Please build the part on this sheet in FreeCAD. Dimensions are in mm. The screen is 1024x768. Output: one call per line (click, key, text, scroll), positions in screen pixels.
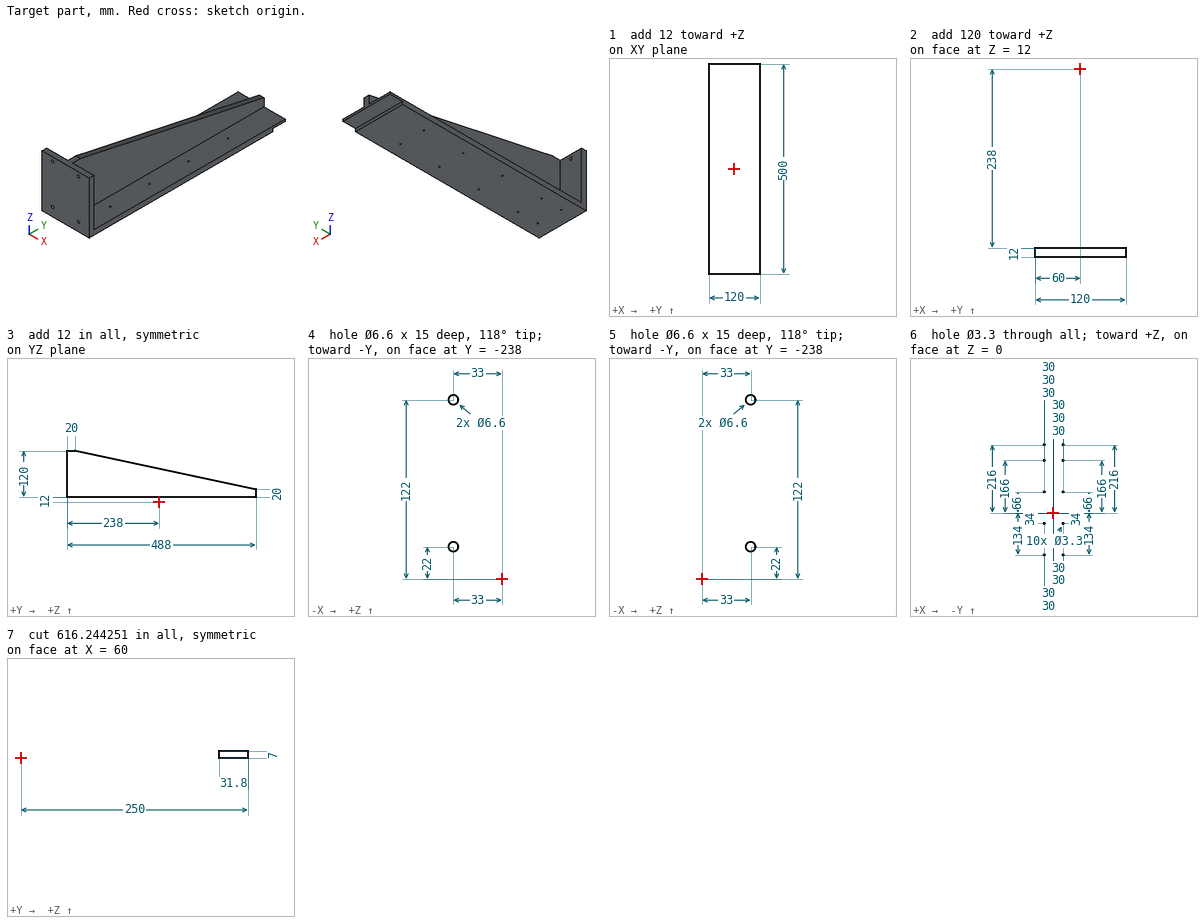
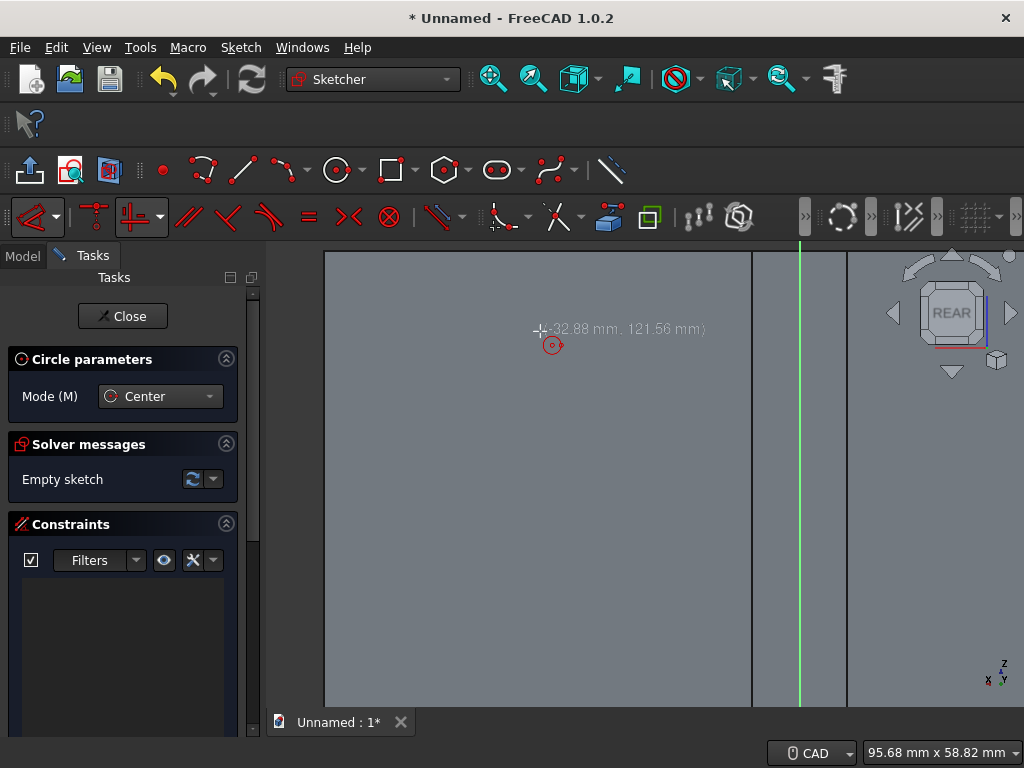
click(538, 330)
click(557, 312)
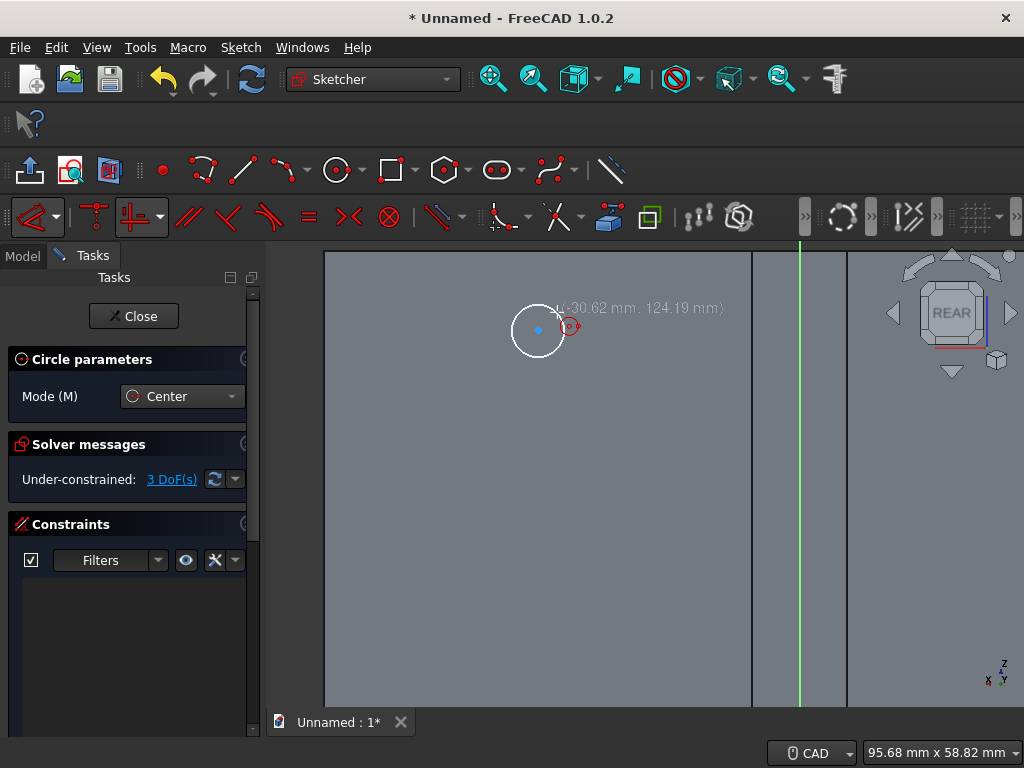
scroll(542, 333, down, 6)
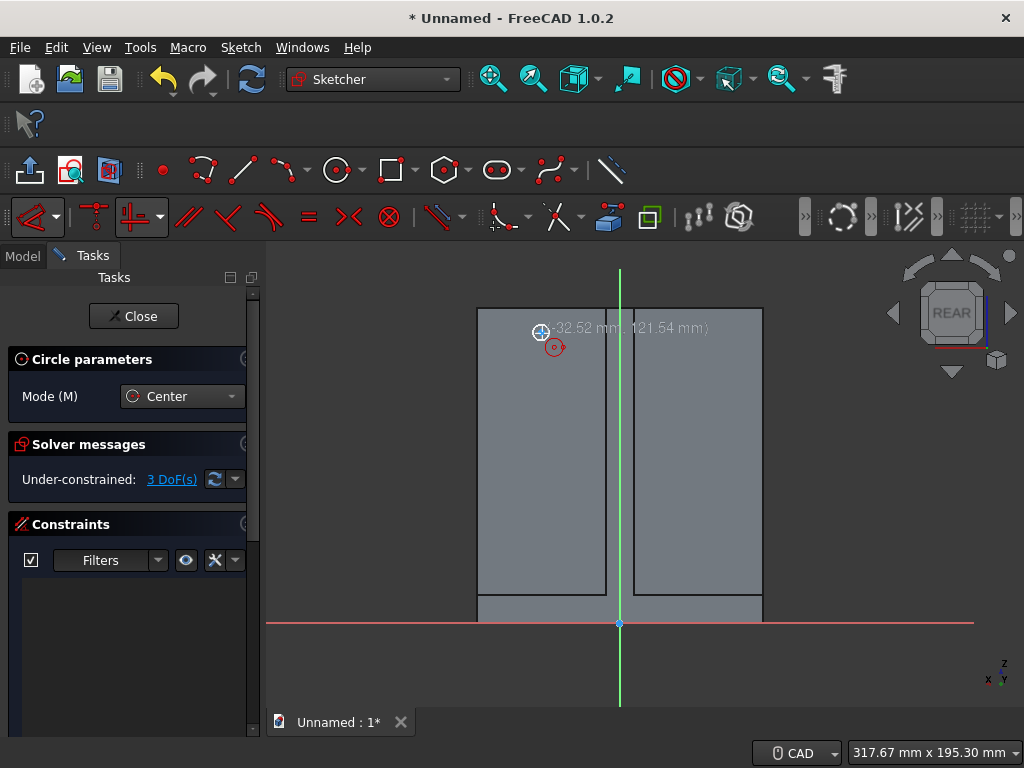
scroll(541, 571, up, 6)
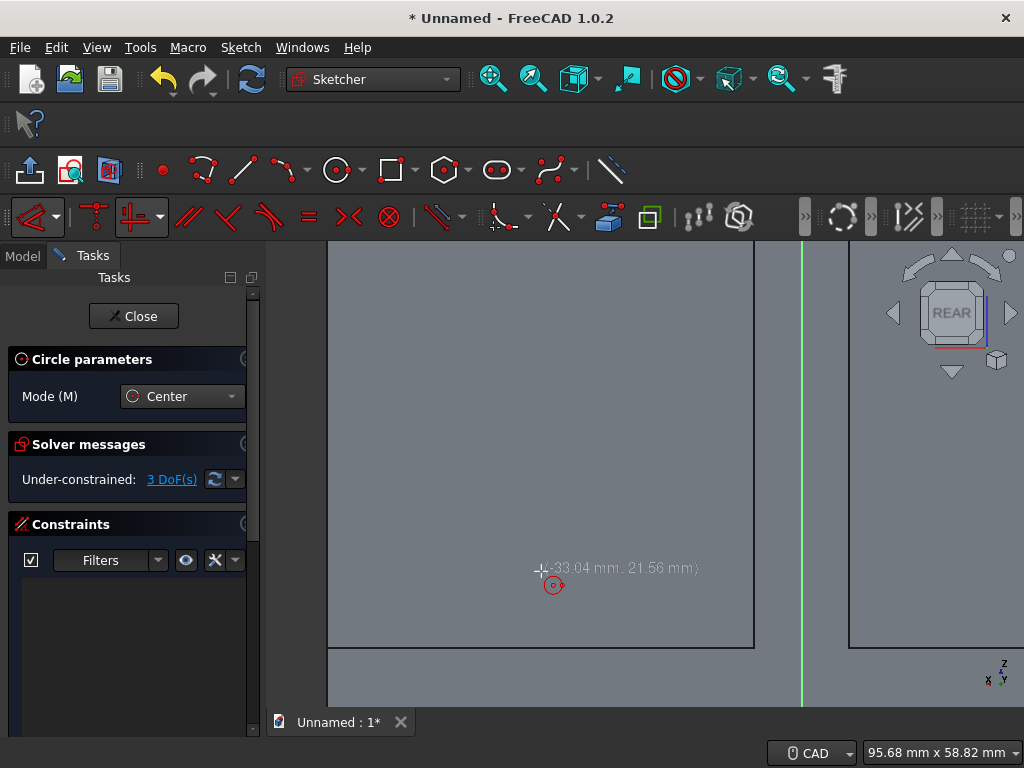
click(540, 569)
click(559, 551)
key(Escape)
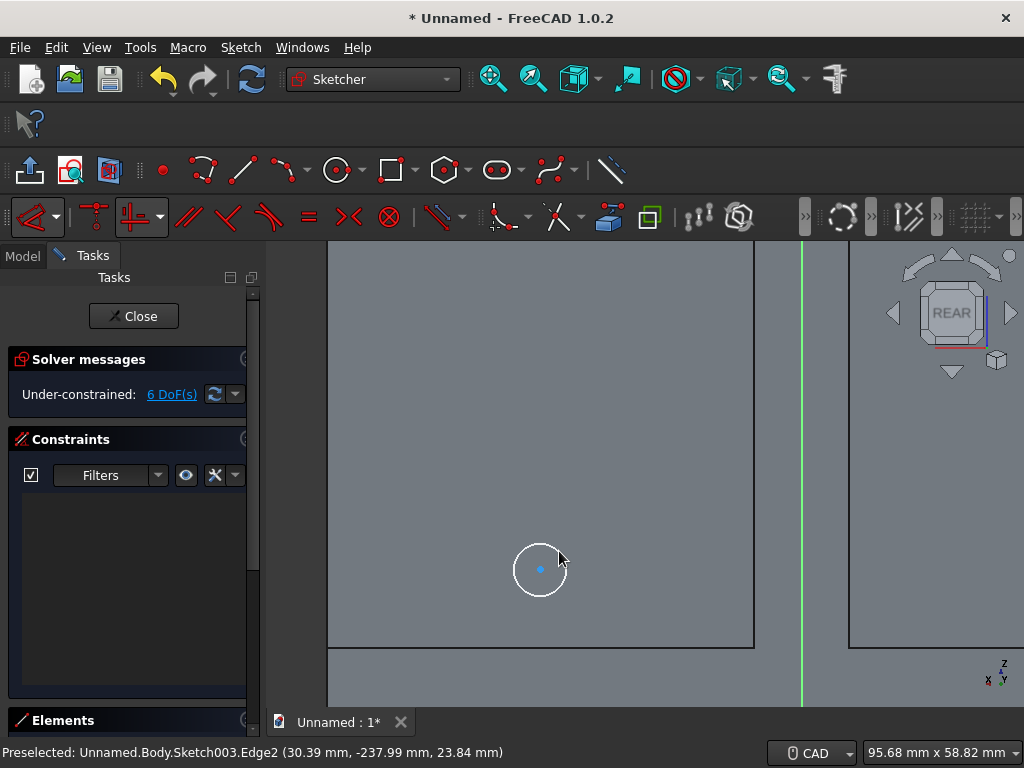
scroll(541, 572, down, 6)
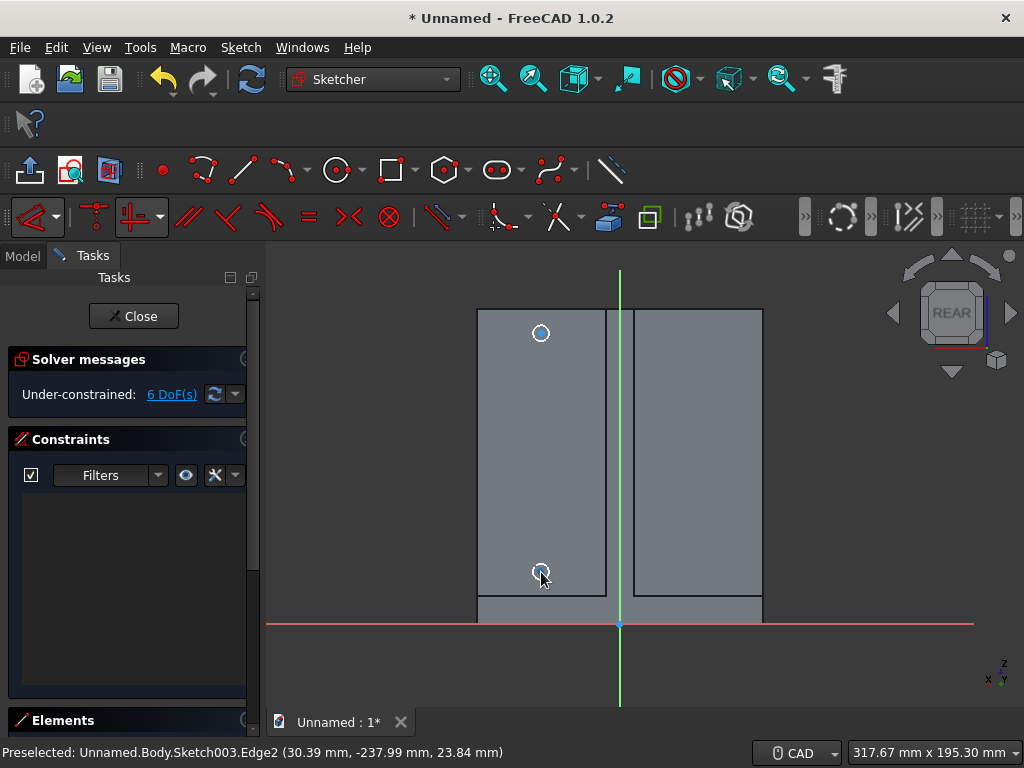
scroll(547, 328, up, 3)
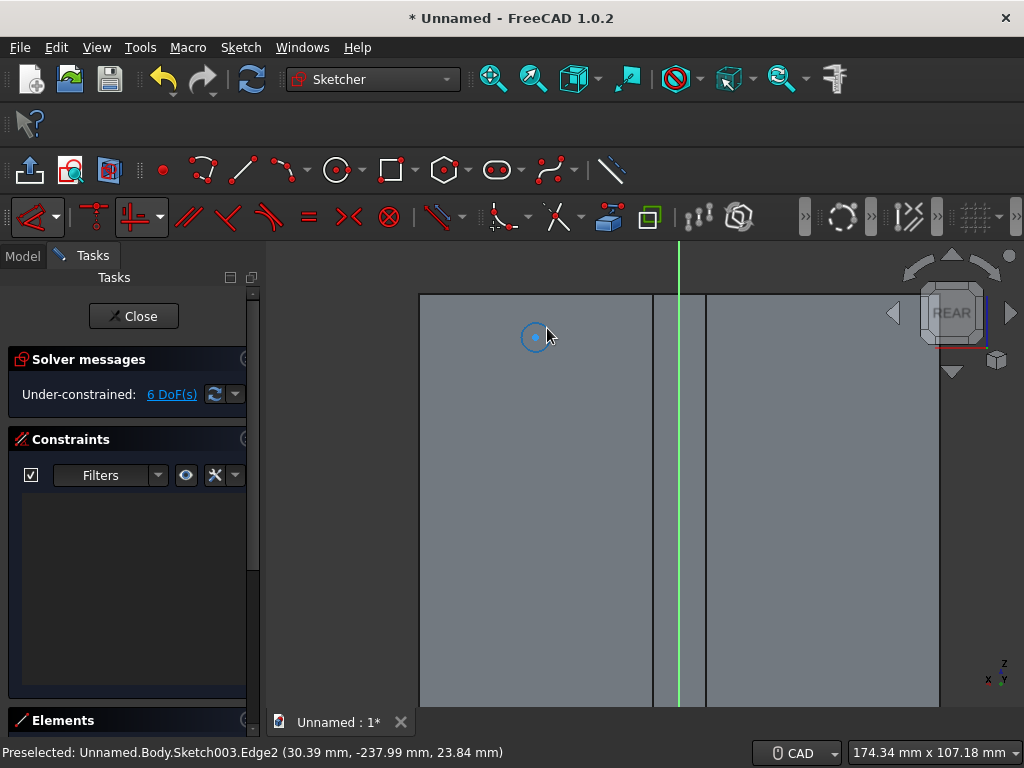
click(546, 327)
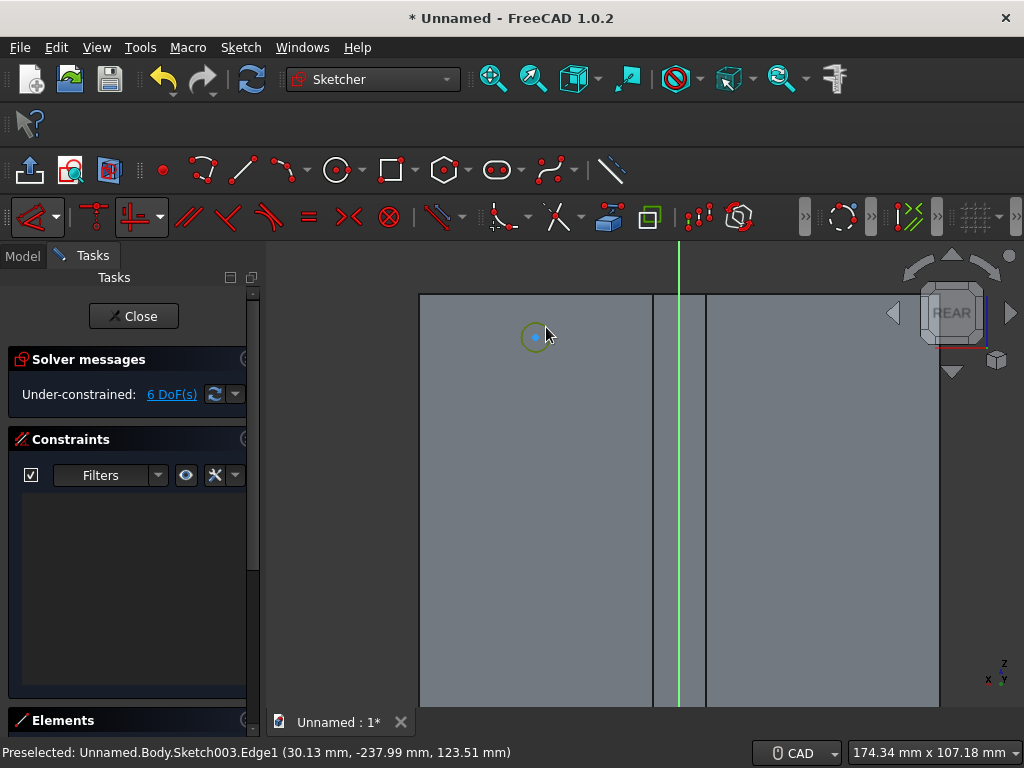
scroll(547, 327, down, 3)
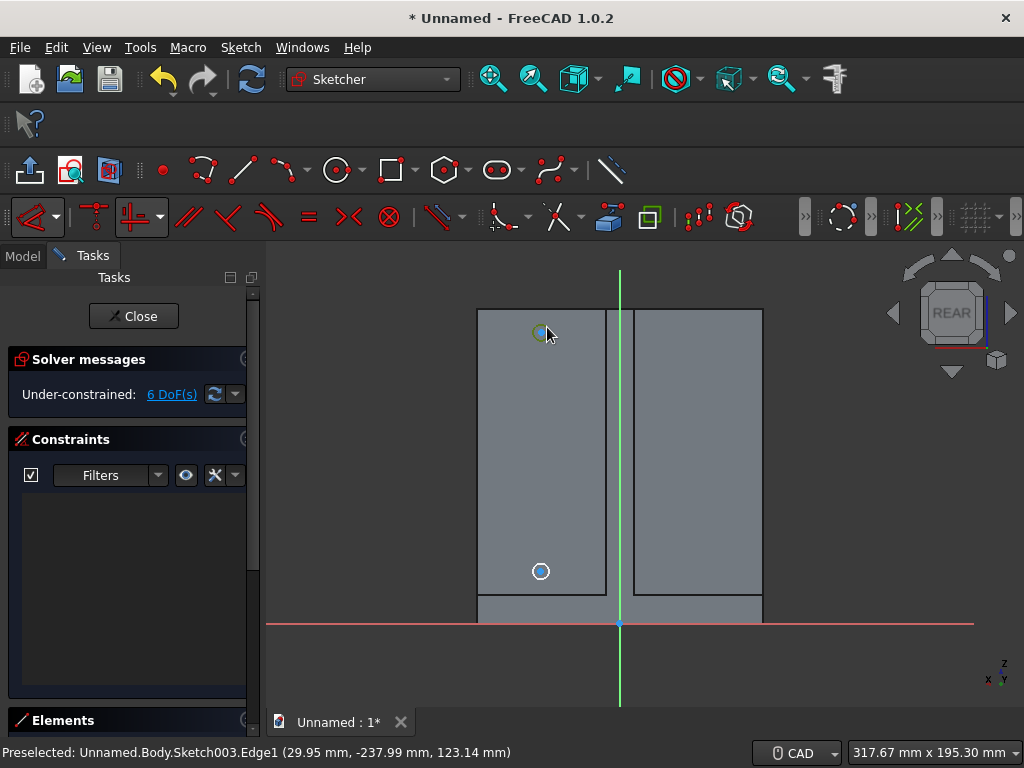
scroll(547, 566, up, 3)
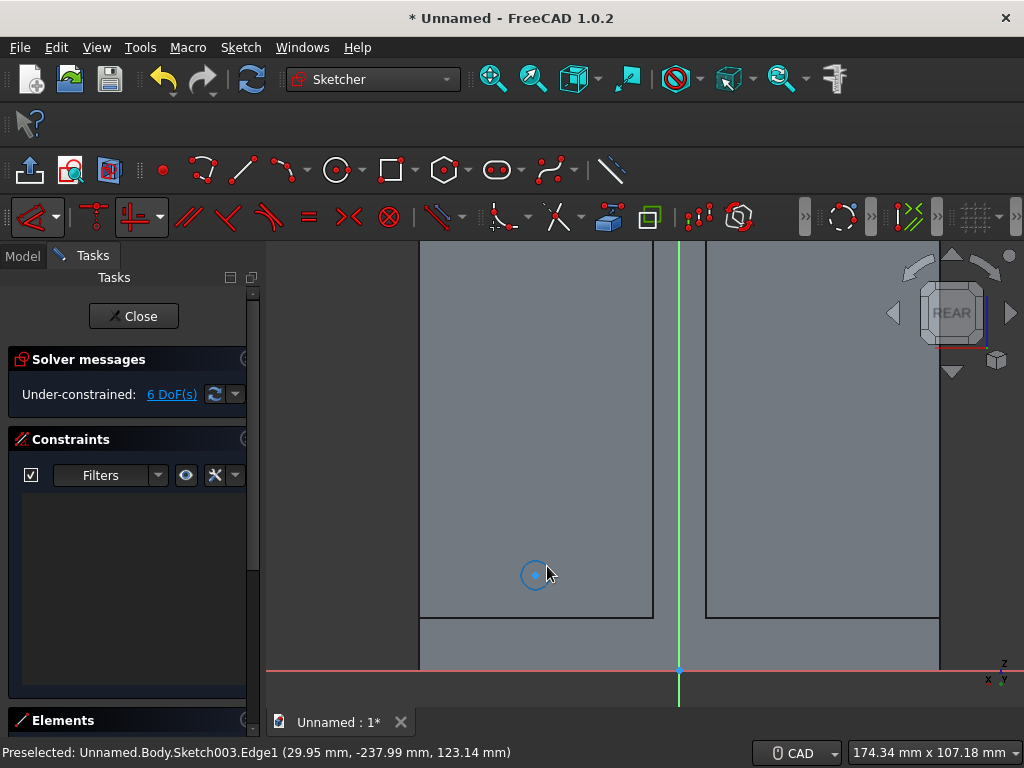
click(546, 565)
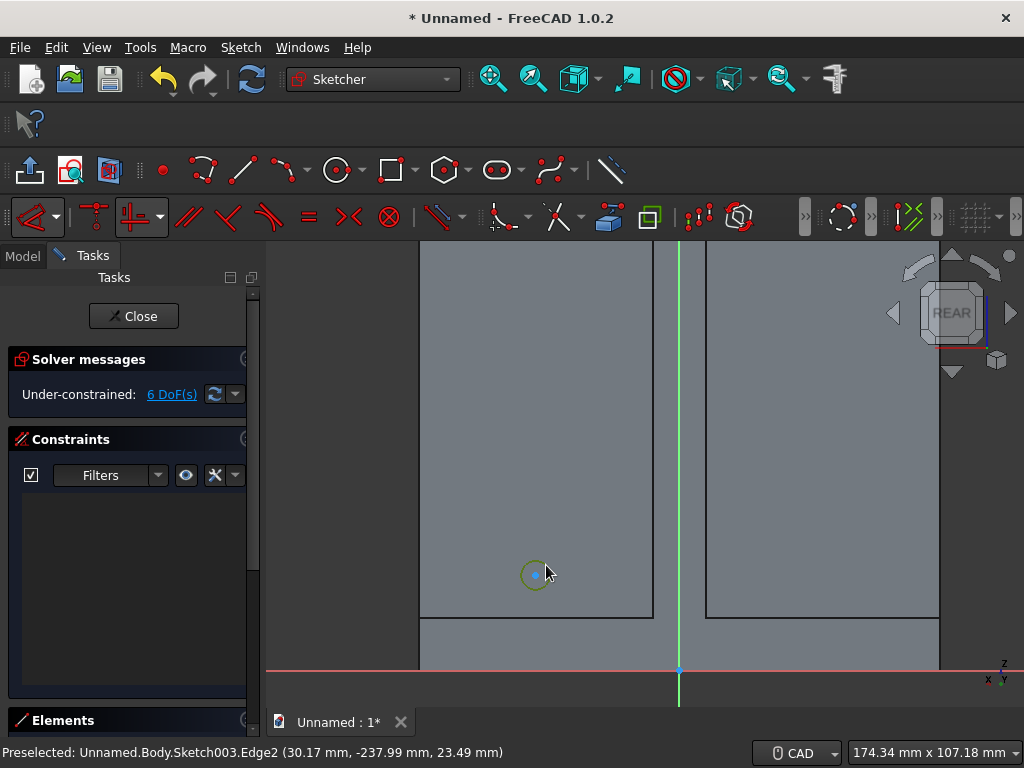
click(310, 218)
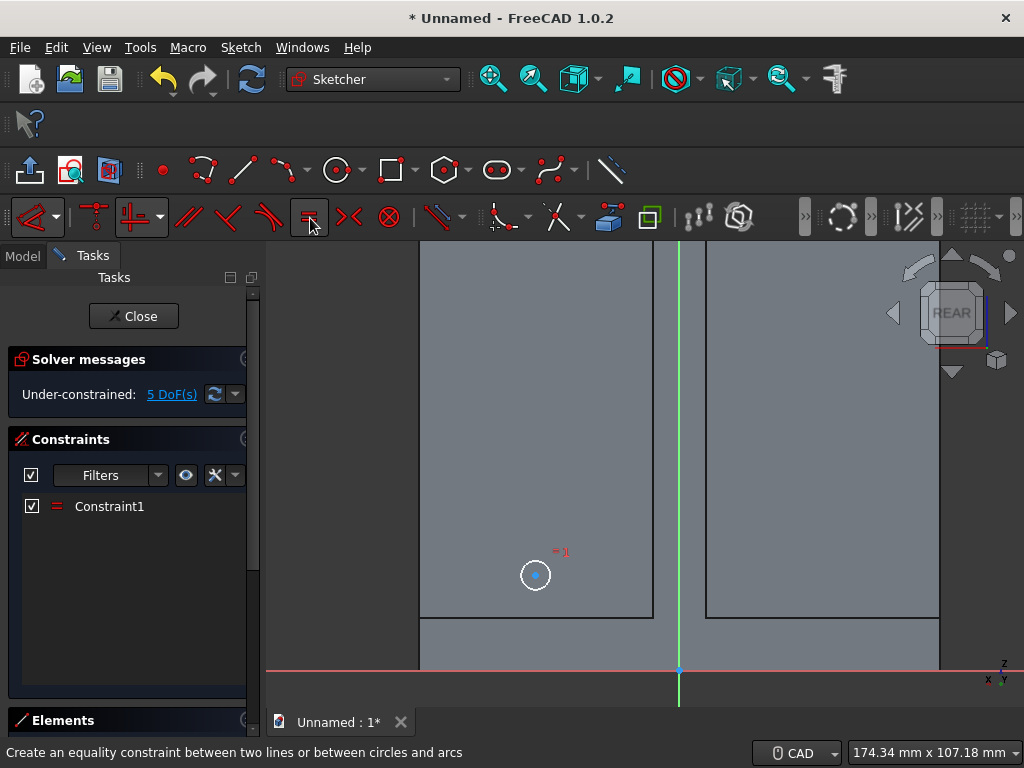
scroll(547, 566, down, 3)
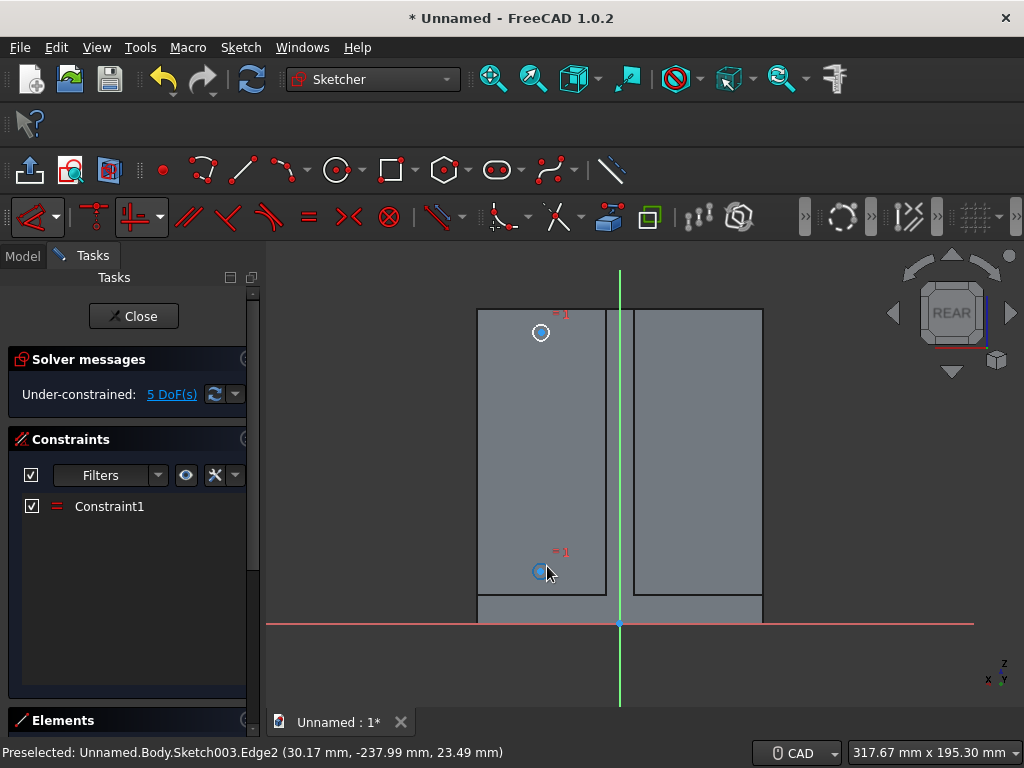
scroll(547, 327, up, 5)